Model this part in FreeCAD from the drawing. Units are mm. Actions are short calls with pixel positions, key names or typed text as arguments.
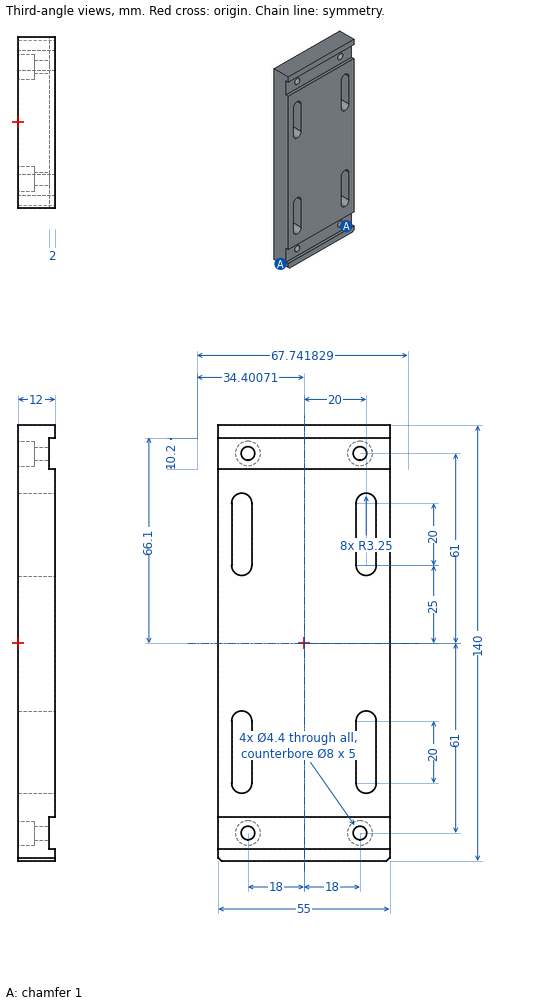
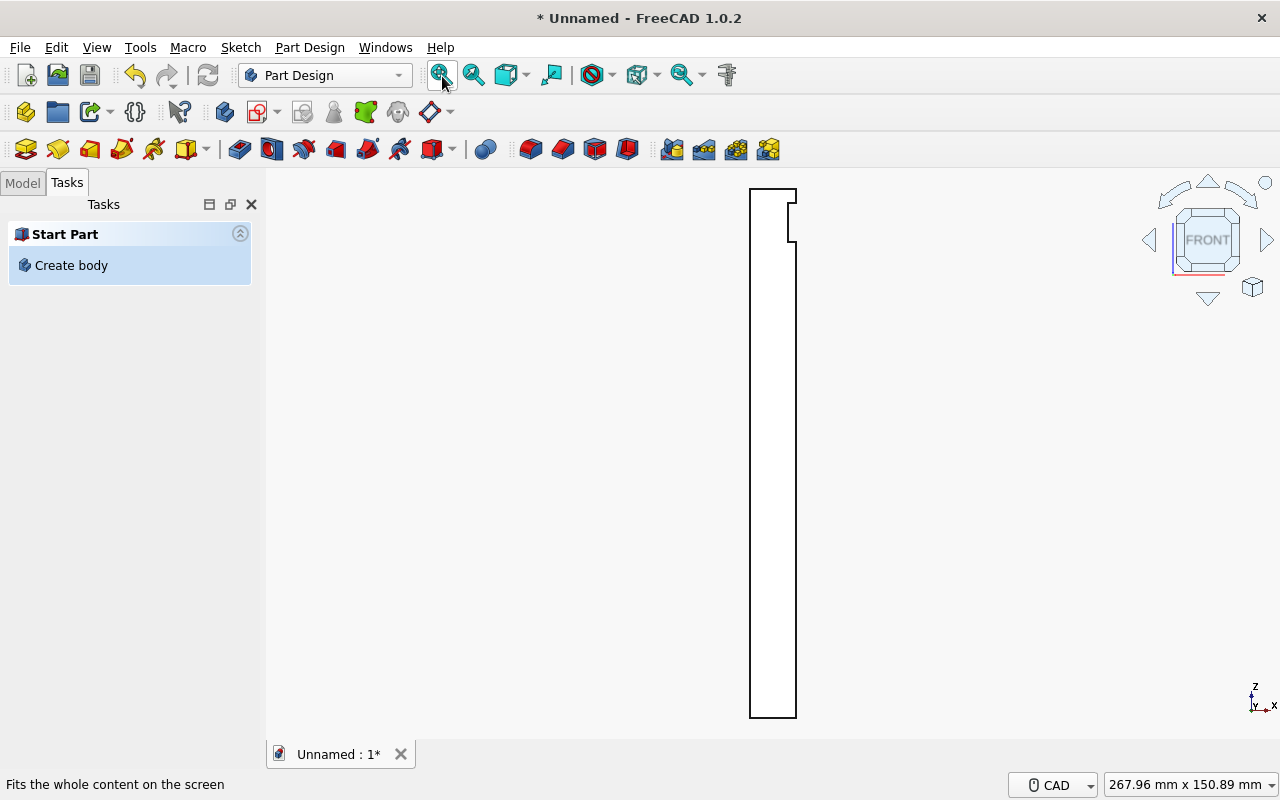
key(3)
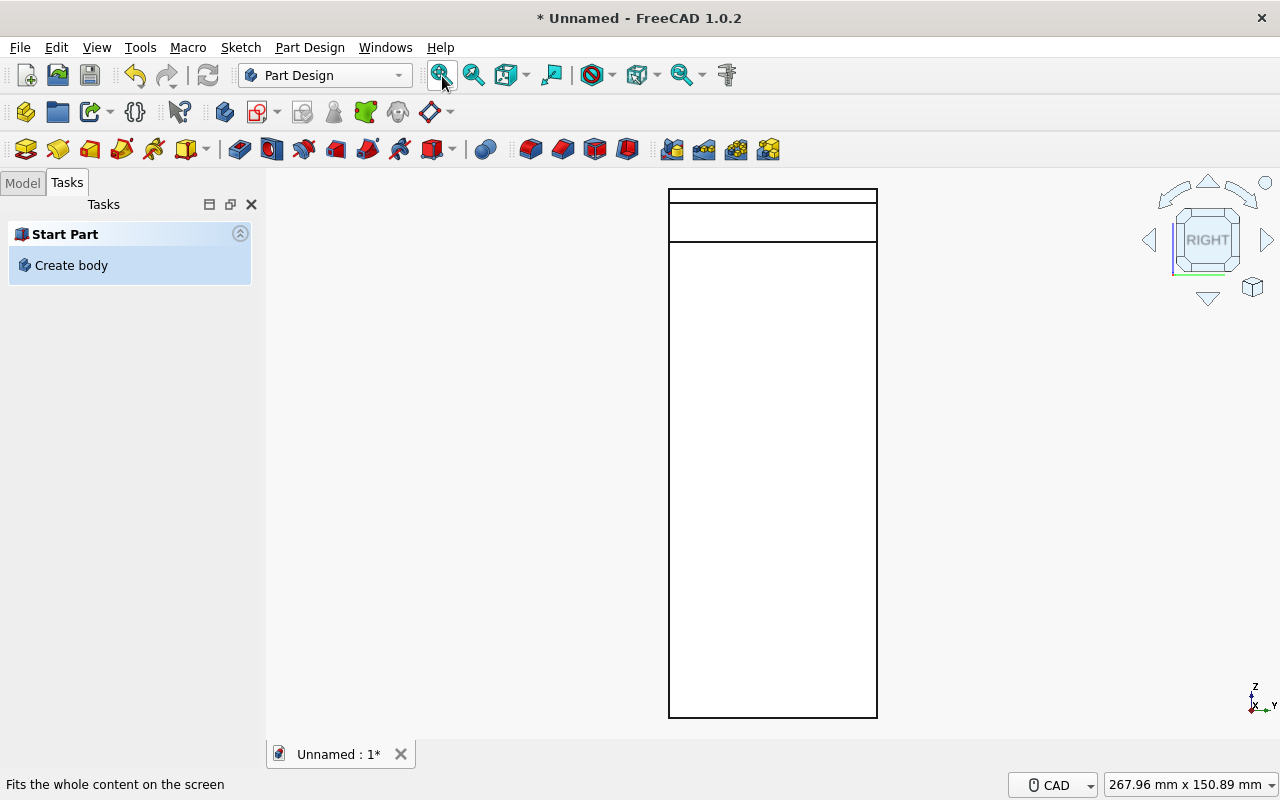
key(5)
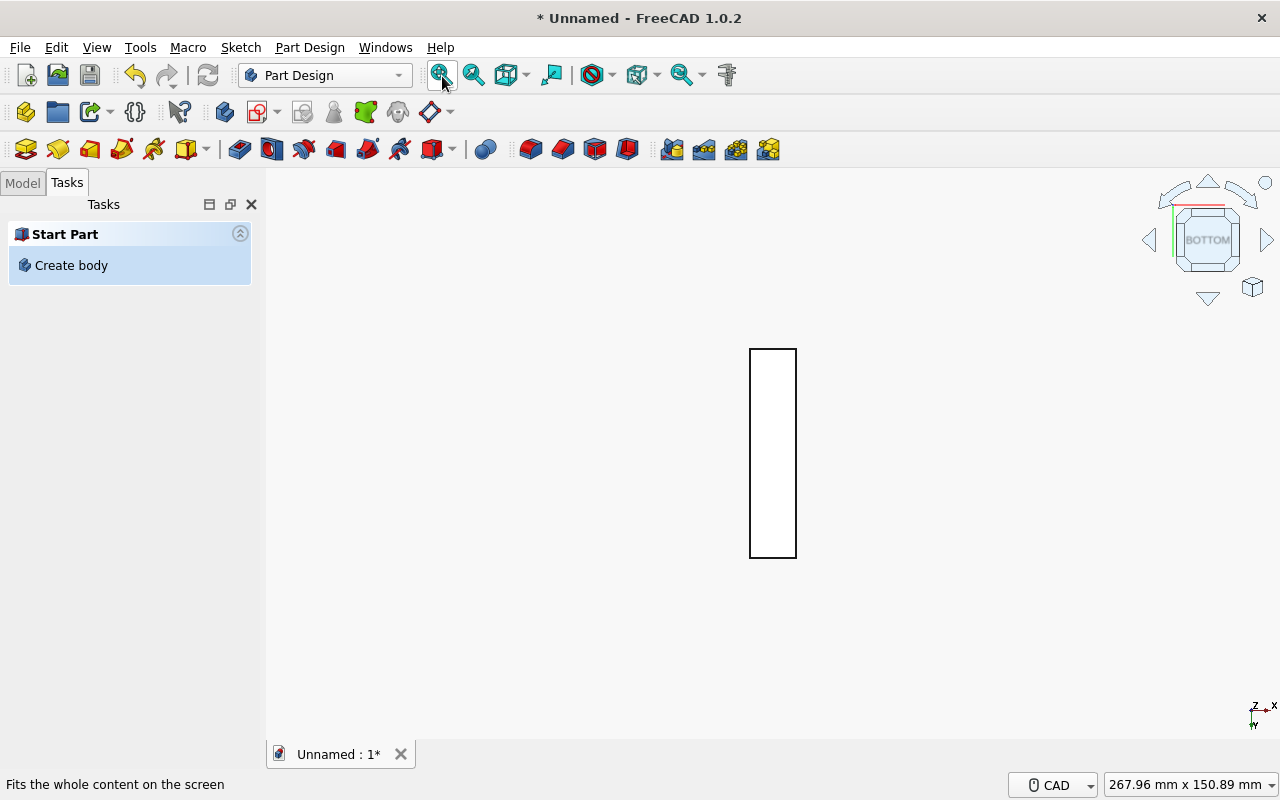
click(442, 76)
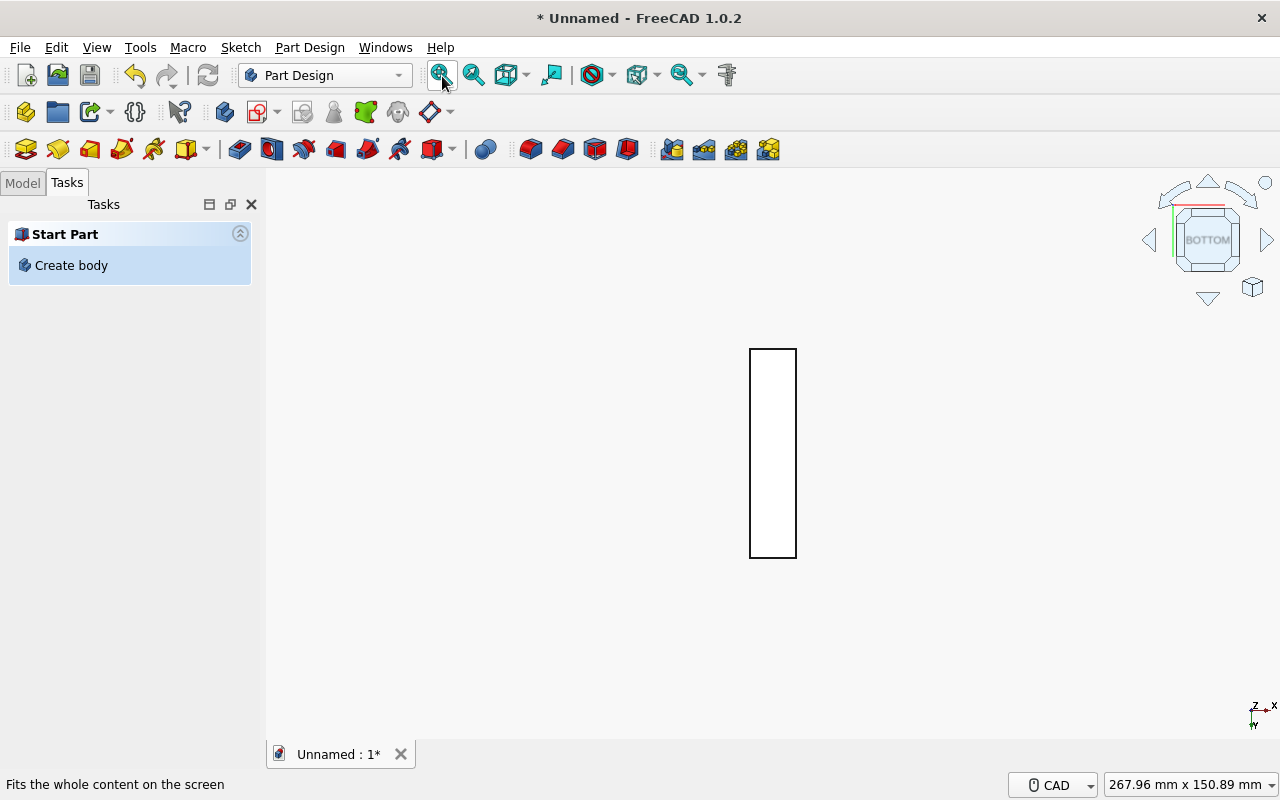
click(773, 348)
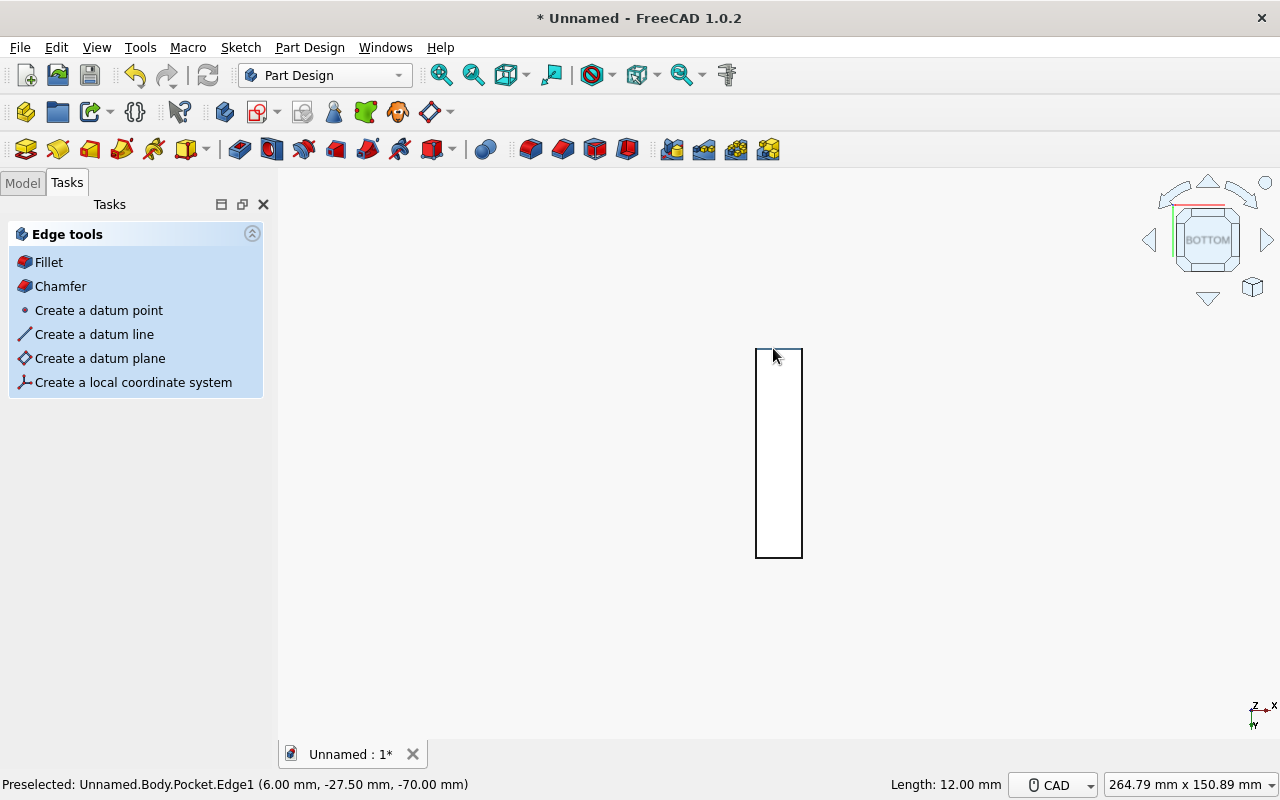
click(779, 557, ctrl)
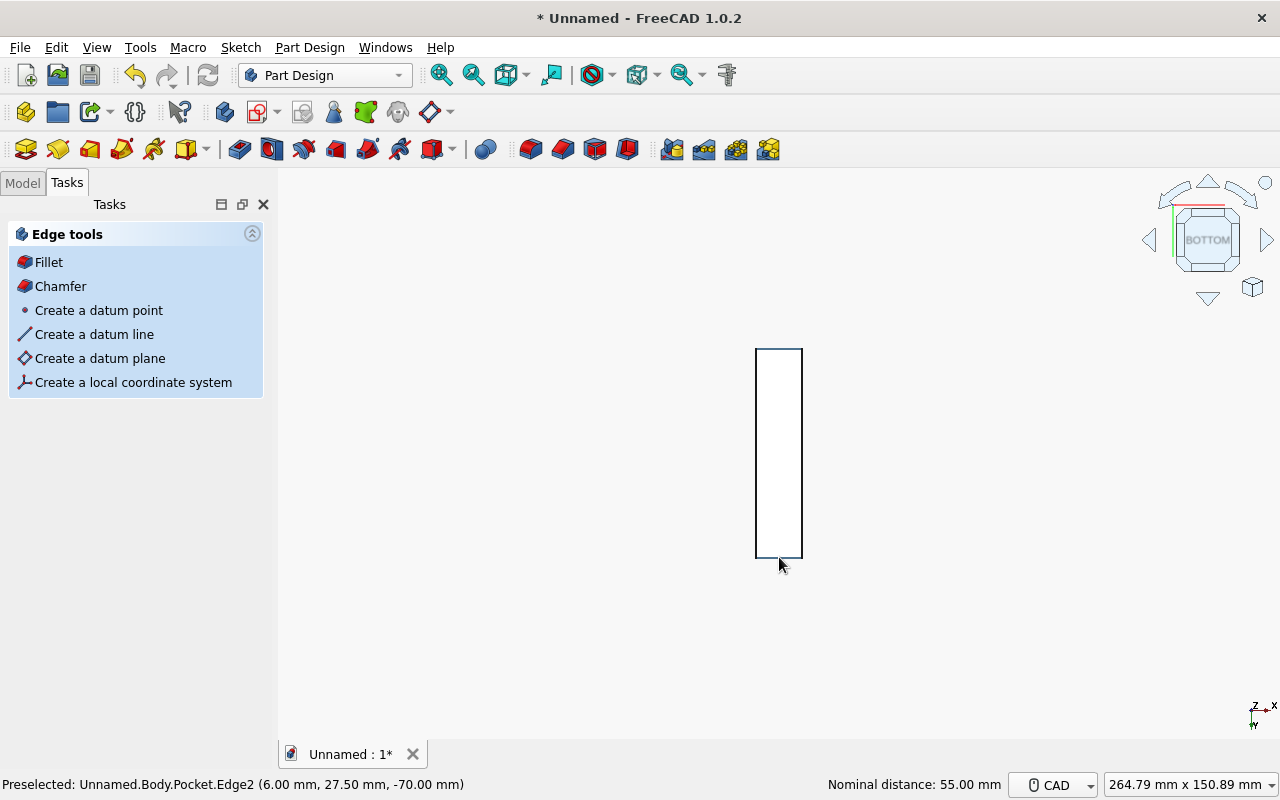
click(564, 150)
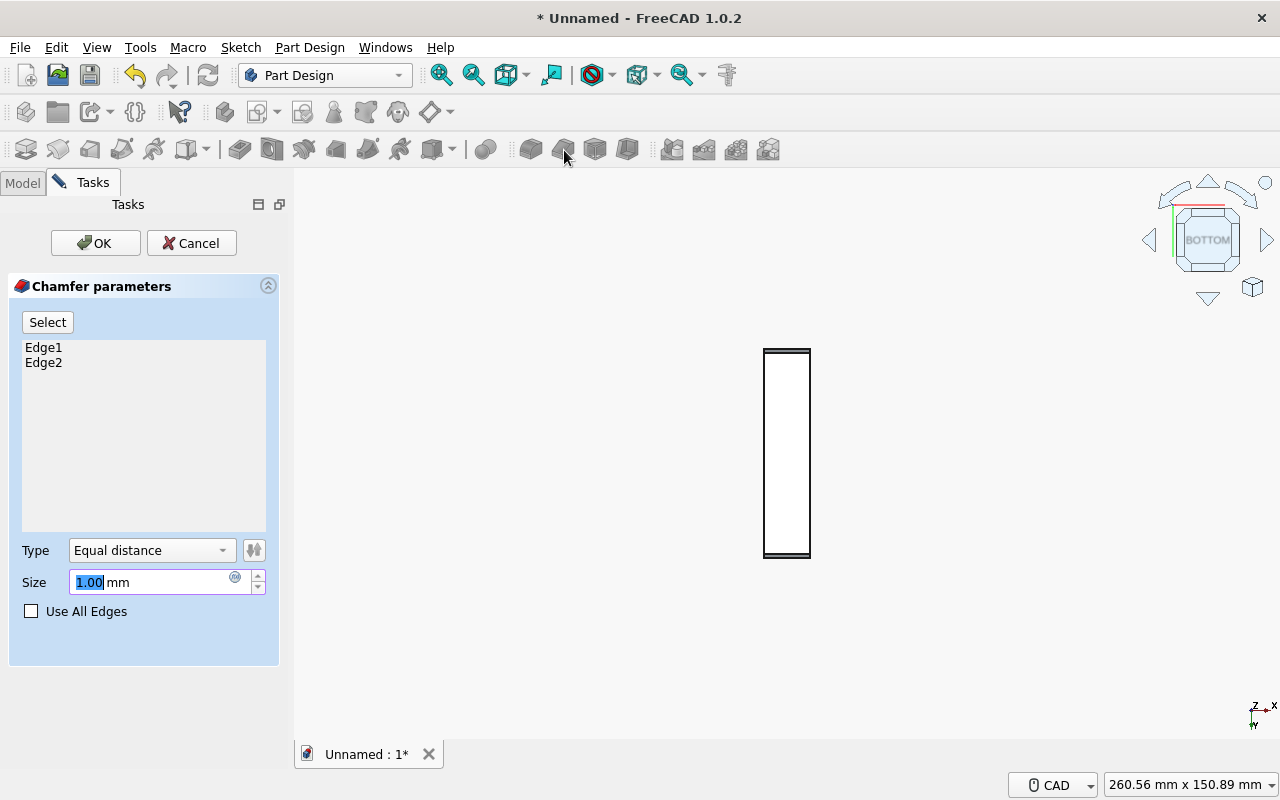
text(1)
key(Tab)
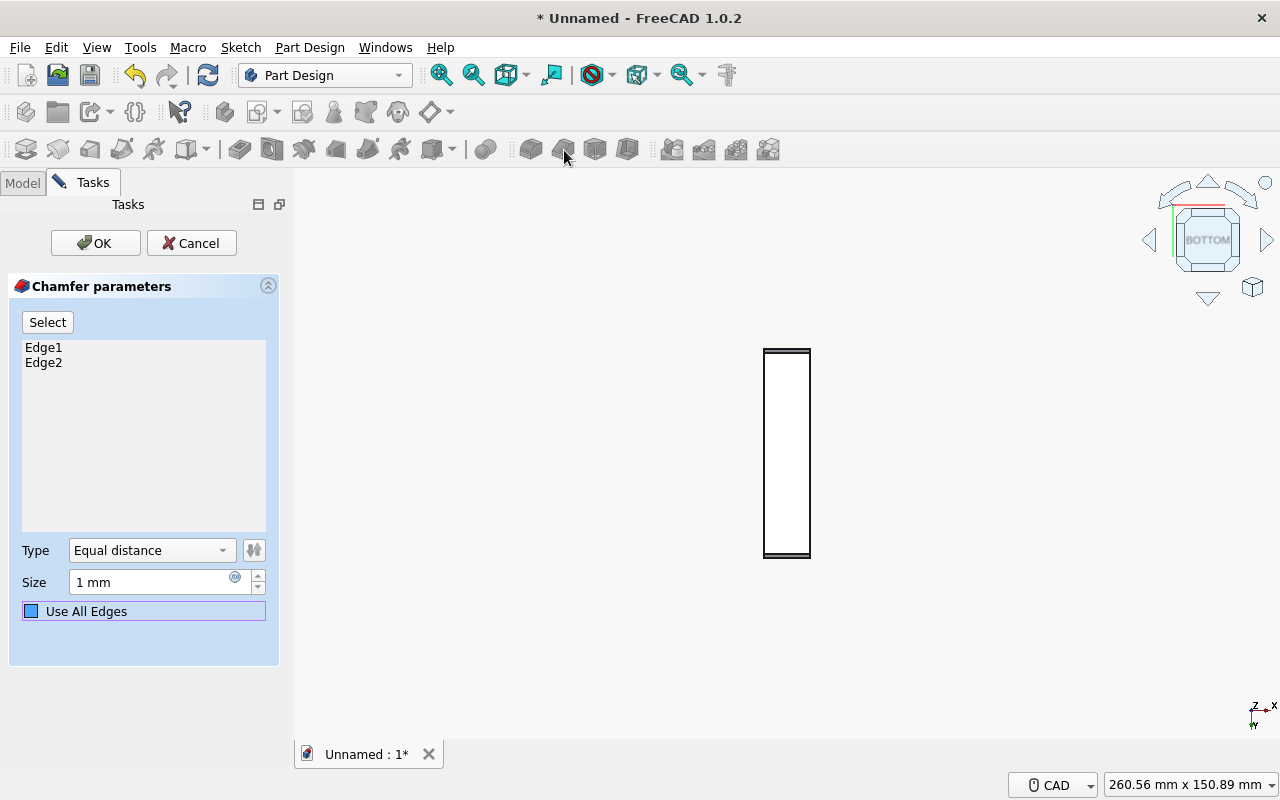
click(96, 243)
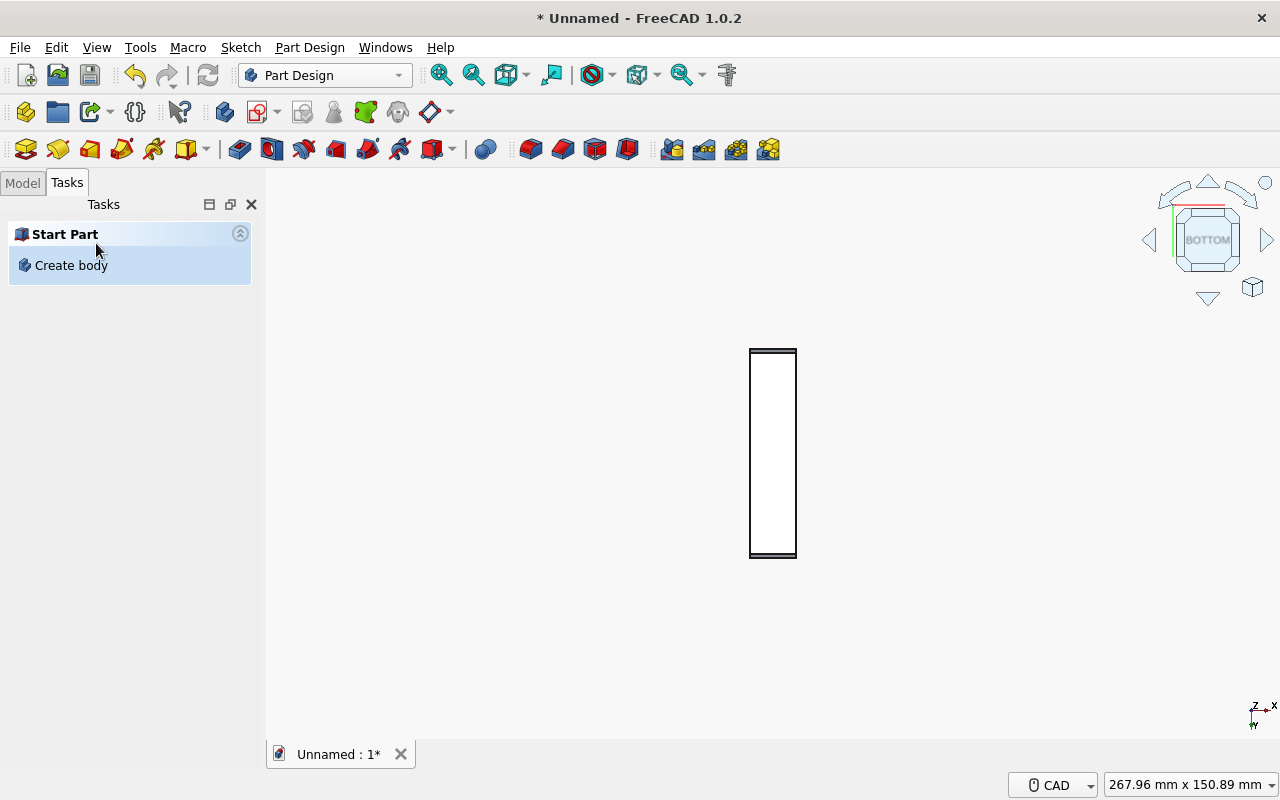
click(442, 76)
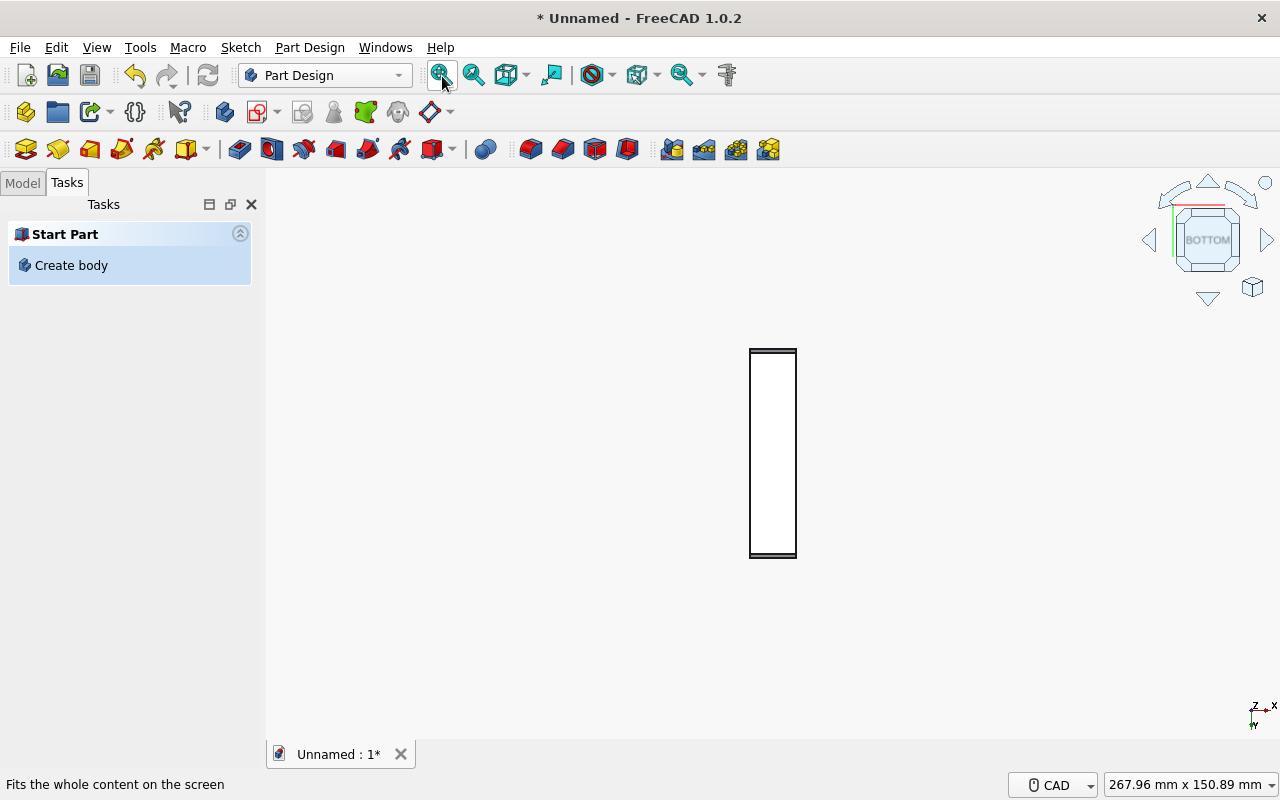
click(23, 182)